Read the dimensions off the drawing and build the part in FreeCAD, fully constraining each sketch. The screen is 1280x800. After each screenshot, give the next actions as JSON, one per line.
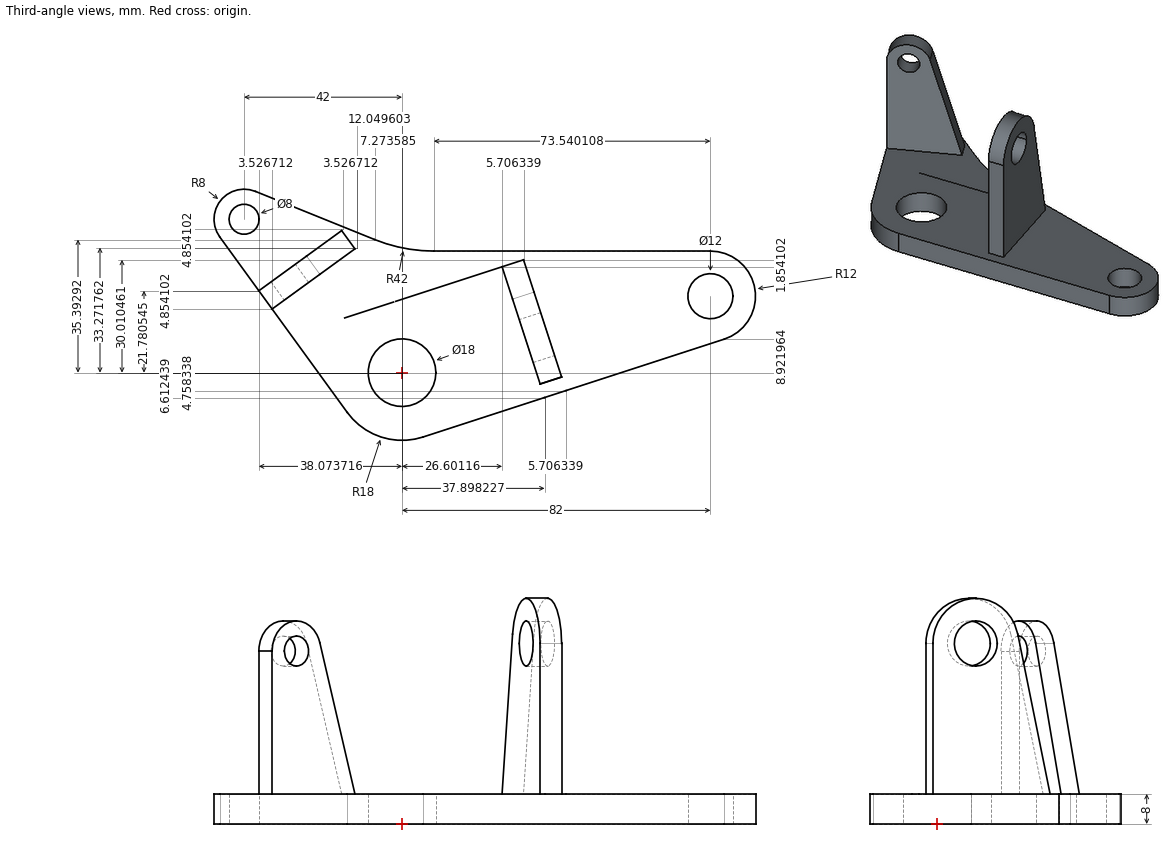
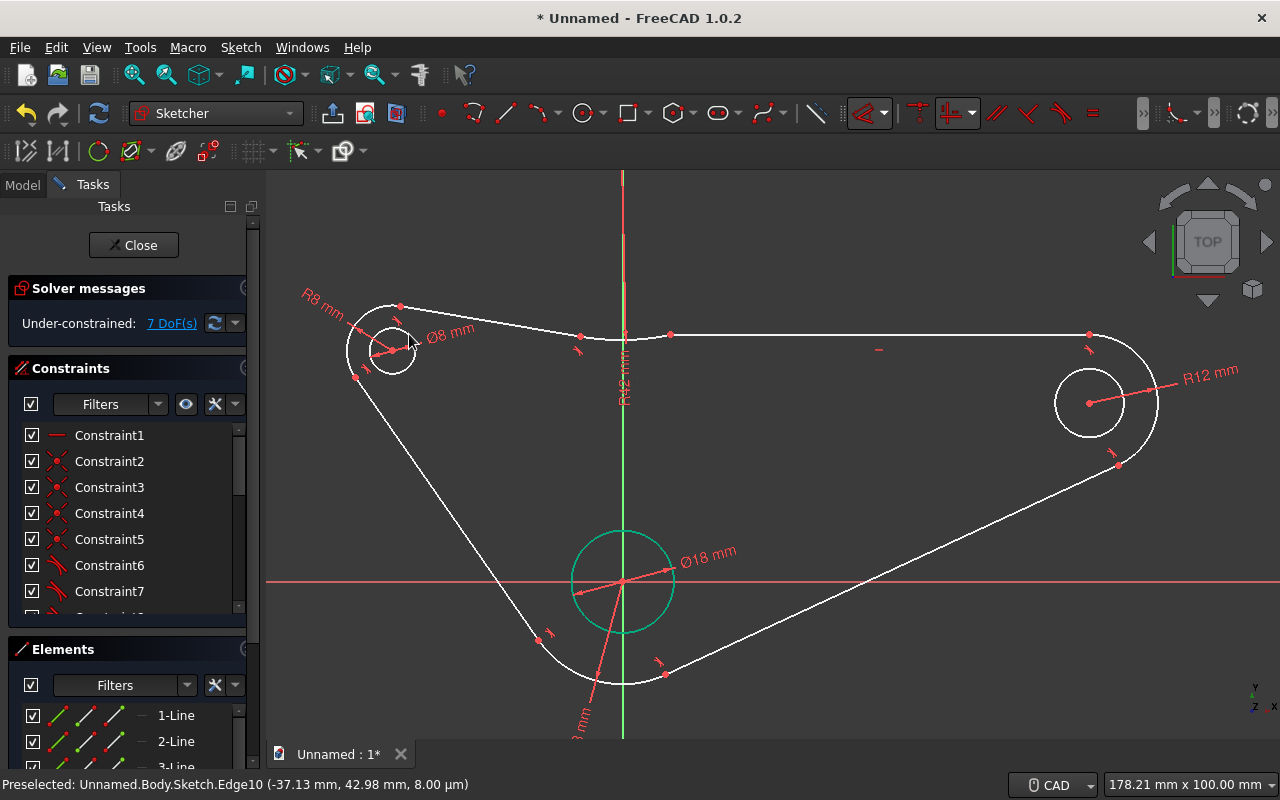
{"action": "left_click", "coordinate": [1114, 379]}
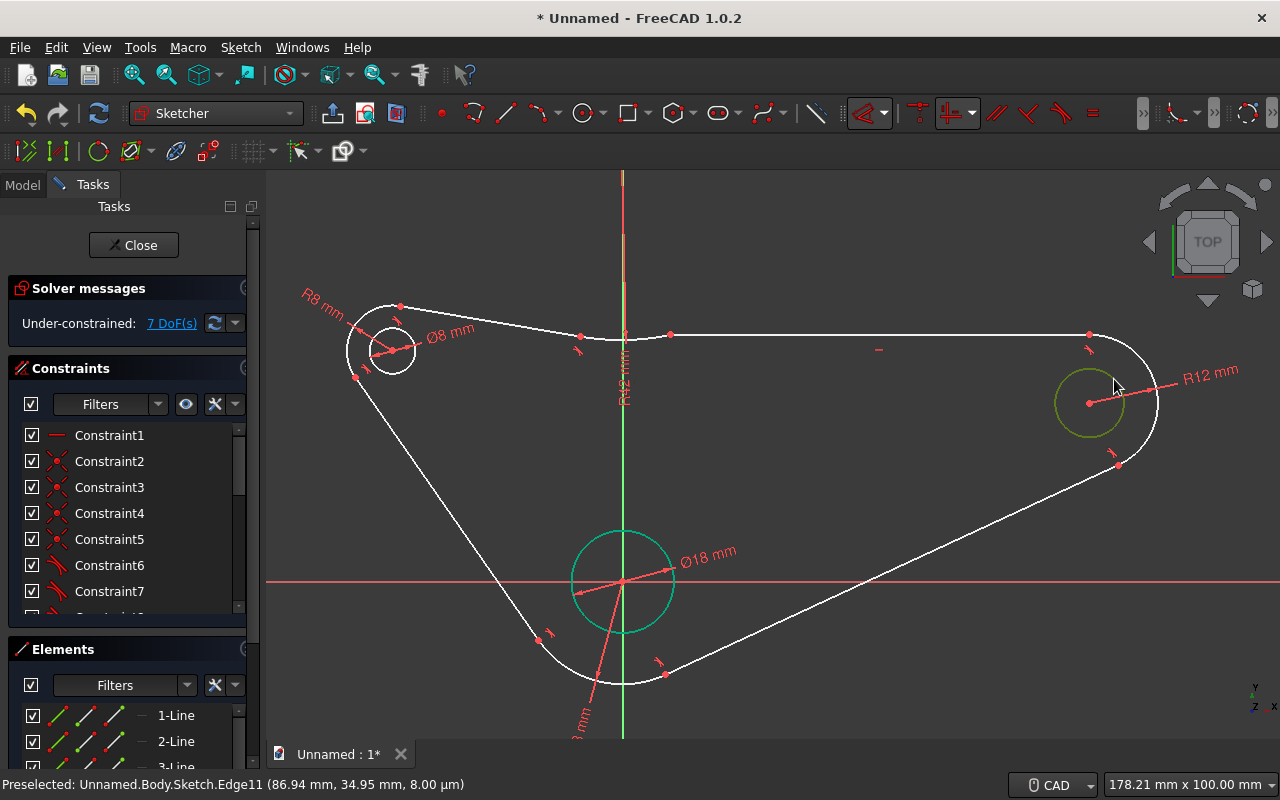
{"action": "key", "text": "k o"}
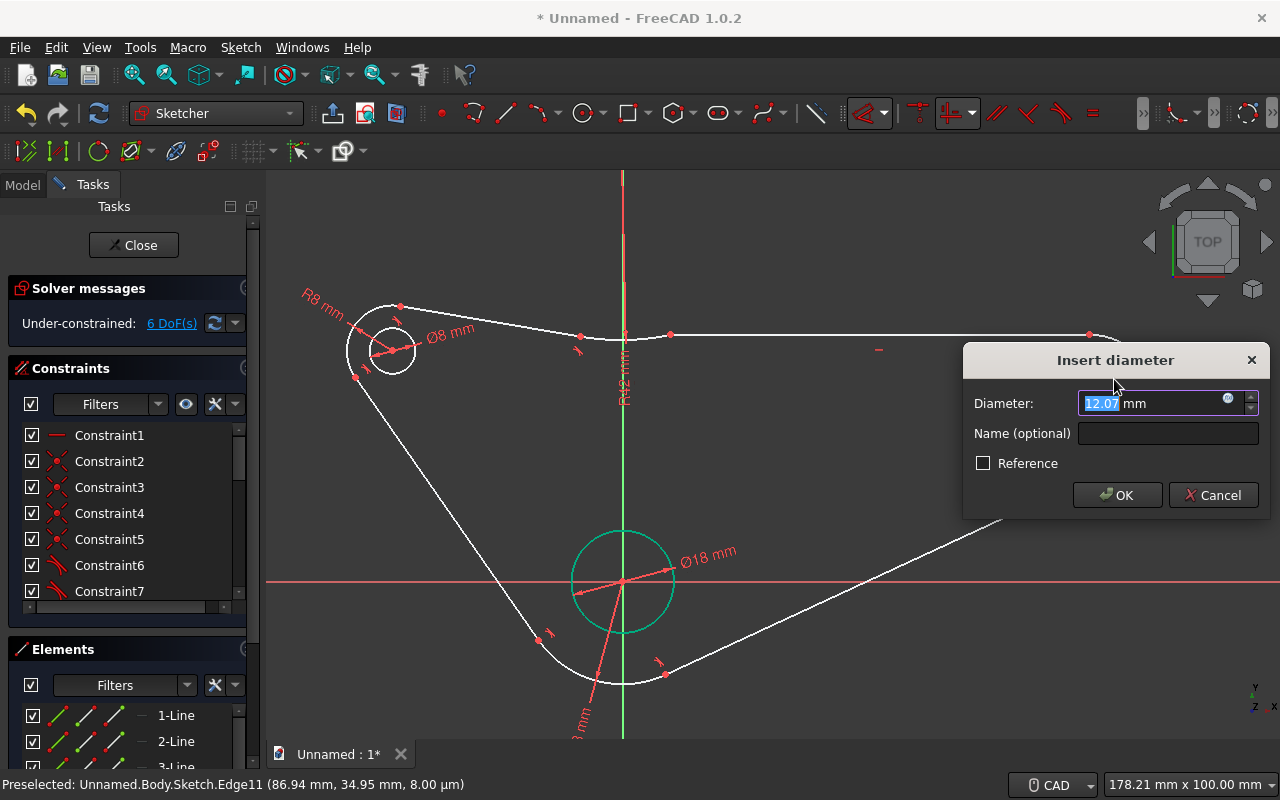
{"action": "type", "text": "12"}
{"action": "key", "text": "Return"}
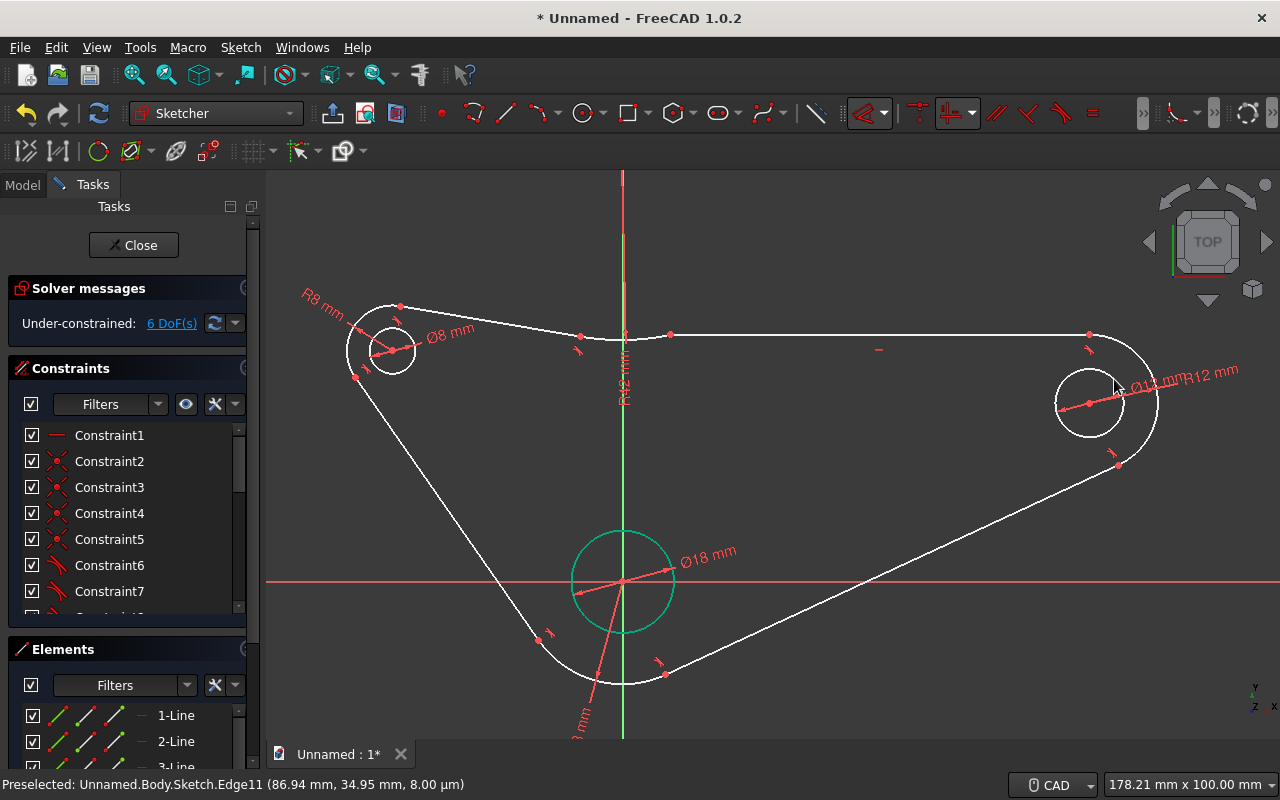
{"action": "left_click", "coordinate": [392, 351]}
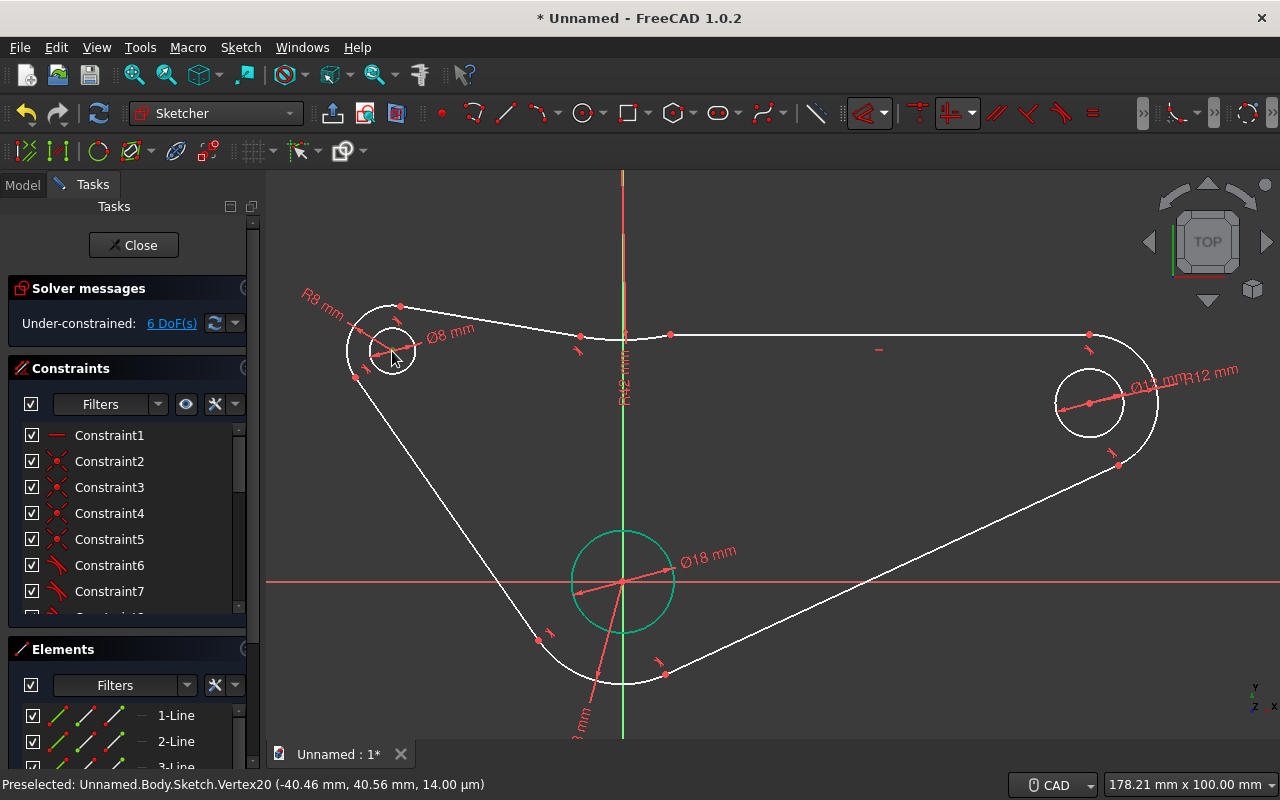
{"action": "key", "text": "l"}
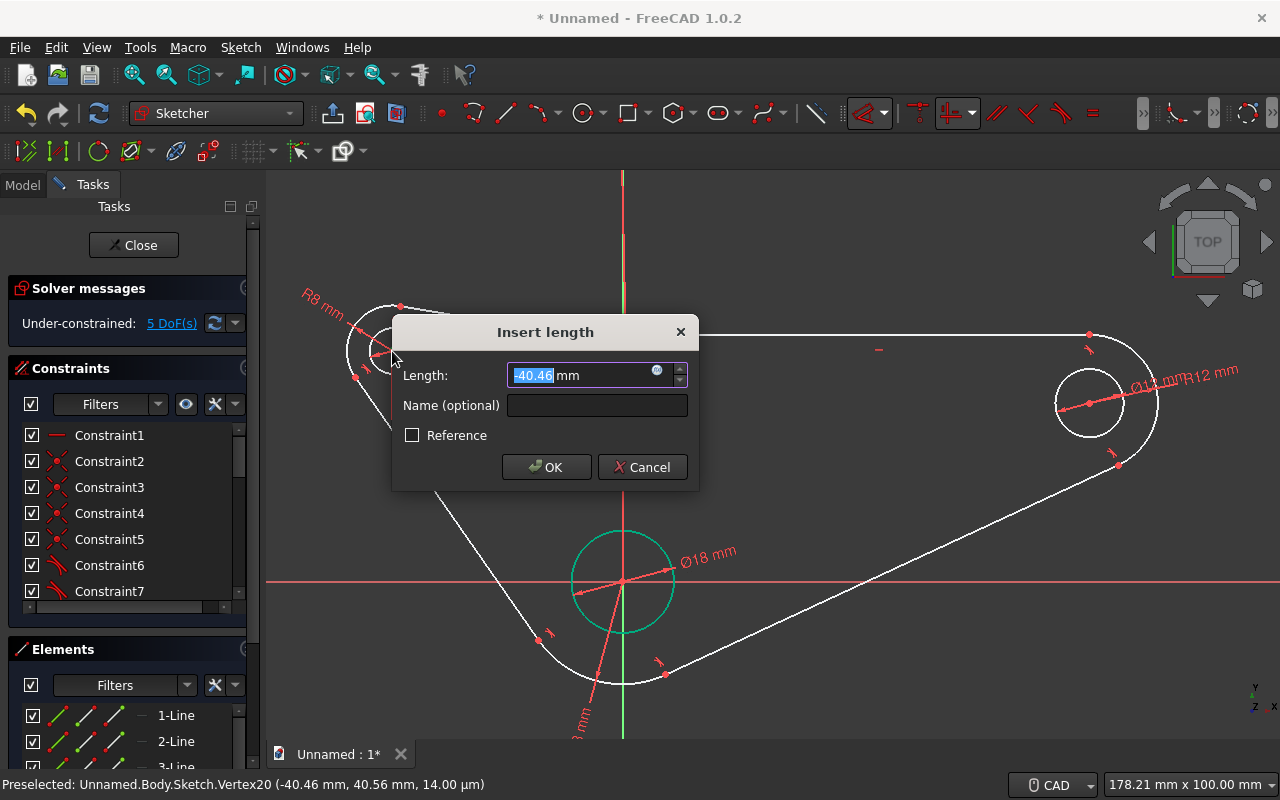
{"action": "type", "text": "-42"}
{"action": "key", "text": "Return"}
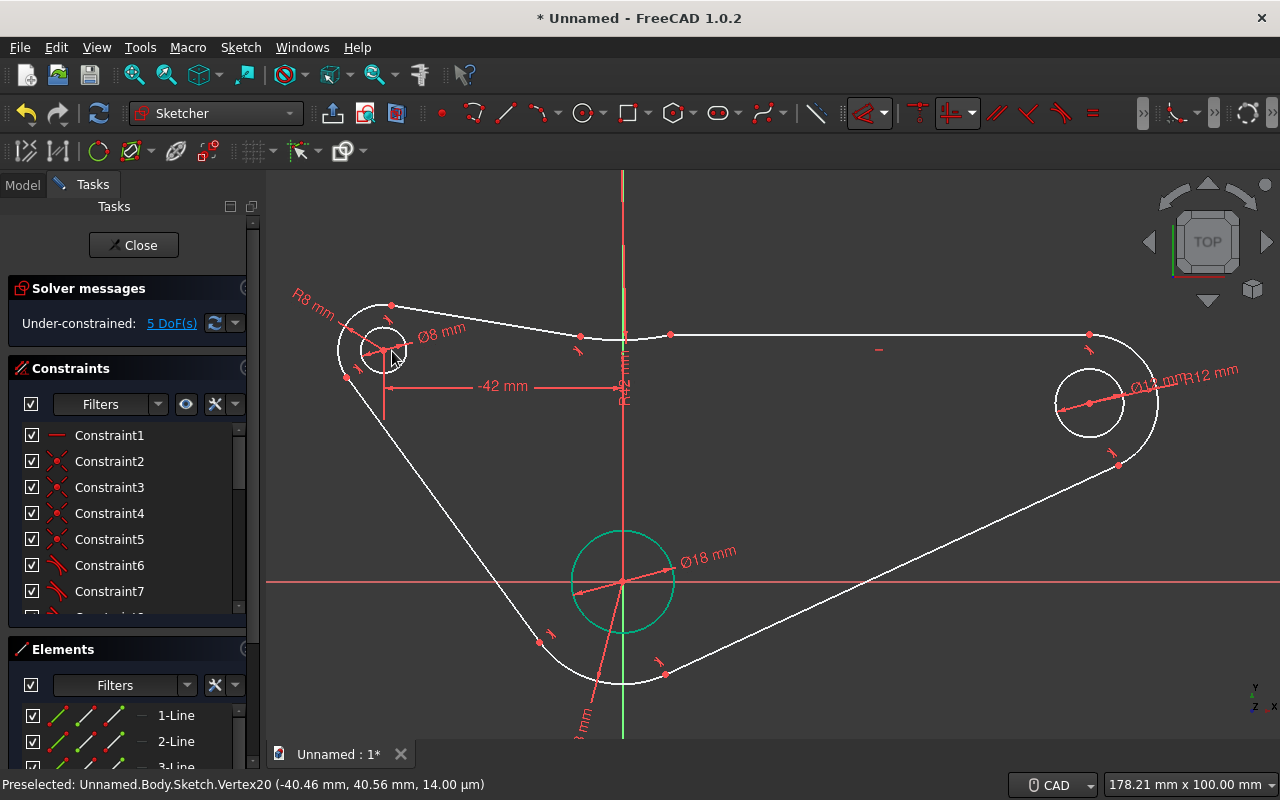
{"action": "left_click", "coordinate": [1090, 403]}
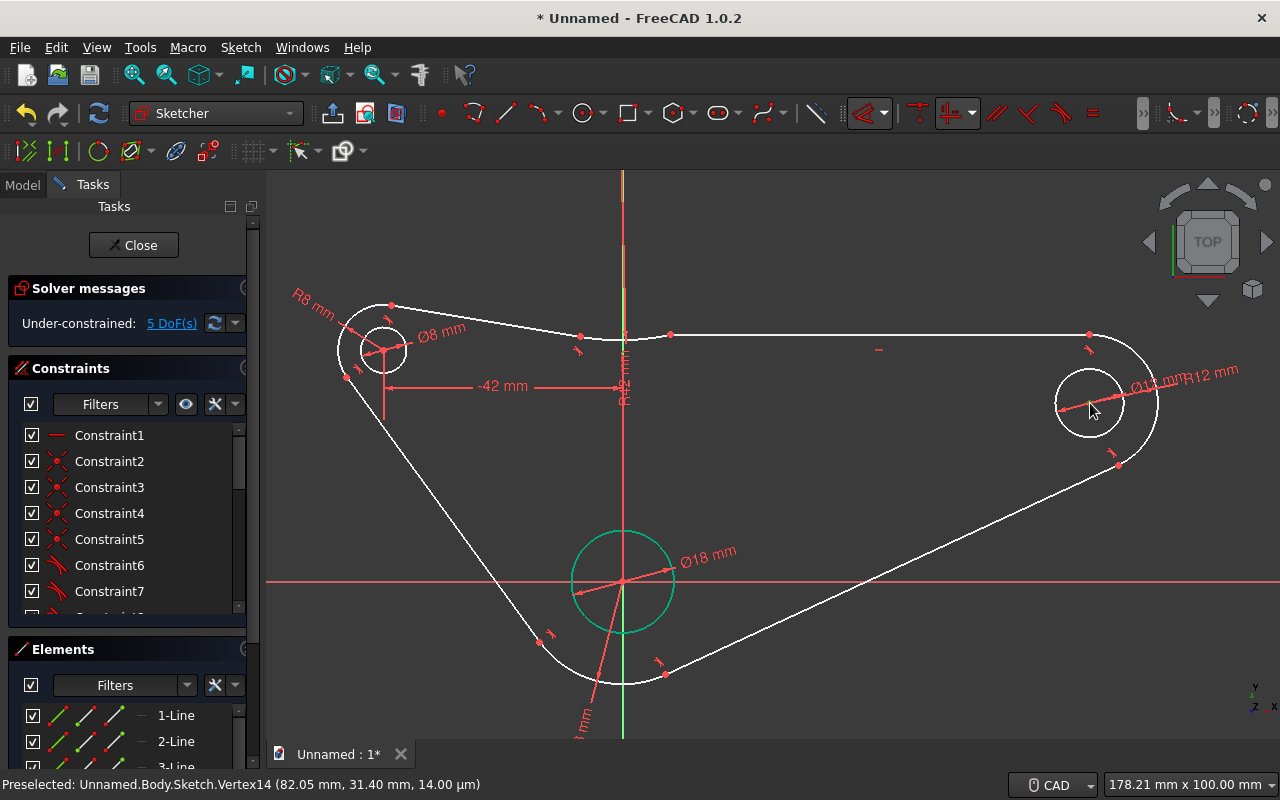
{"action": "key", "text": "l"}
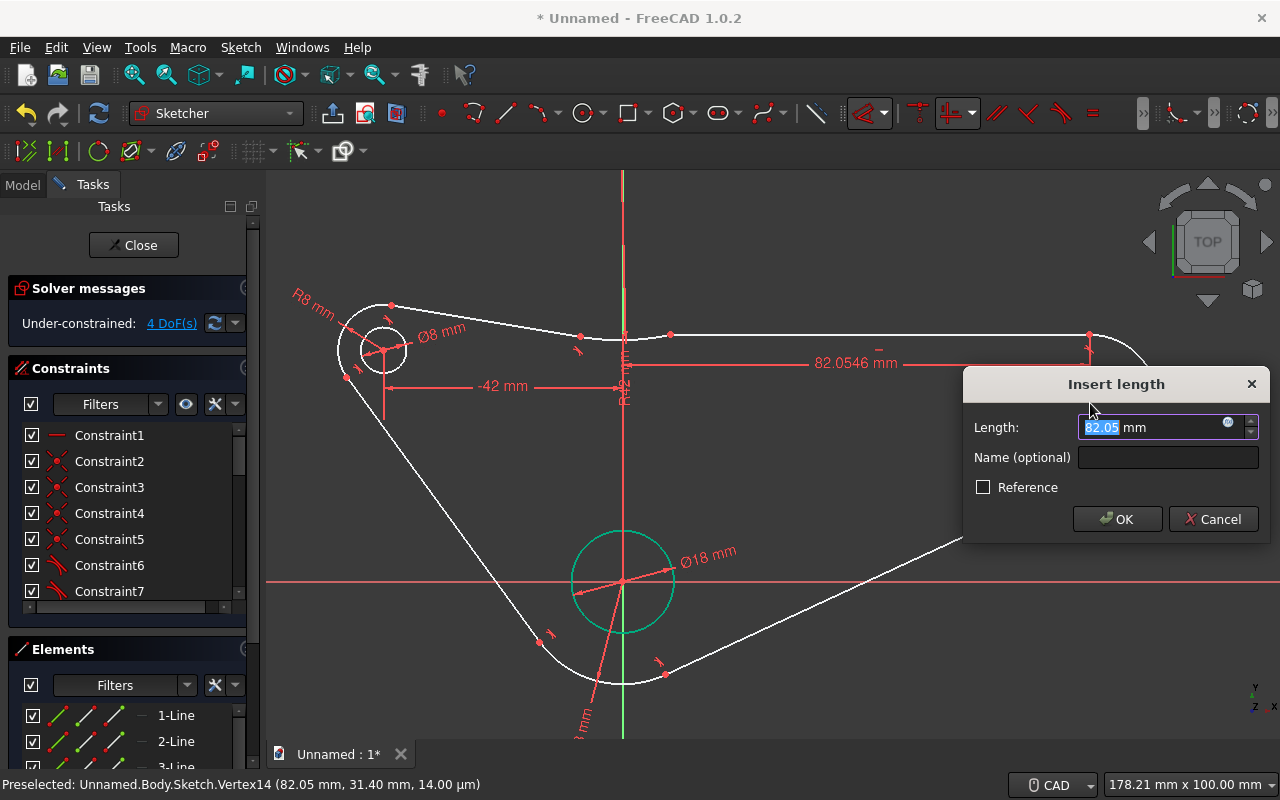
{"action": "type", "text": "82"}
{"action": "key", "text": "Return"}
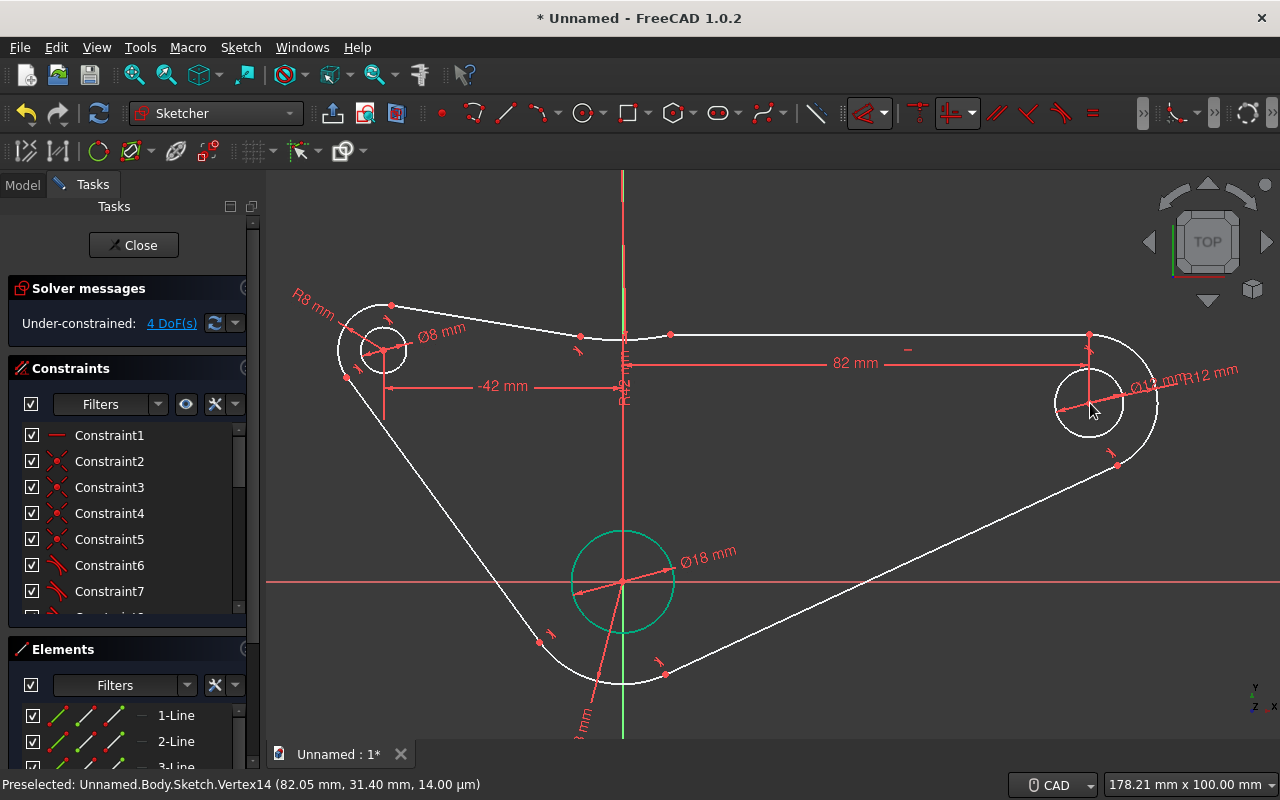
{"action": "left_click", "coordinate": [964, 335]}